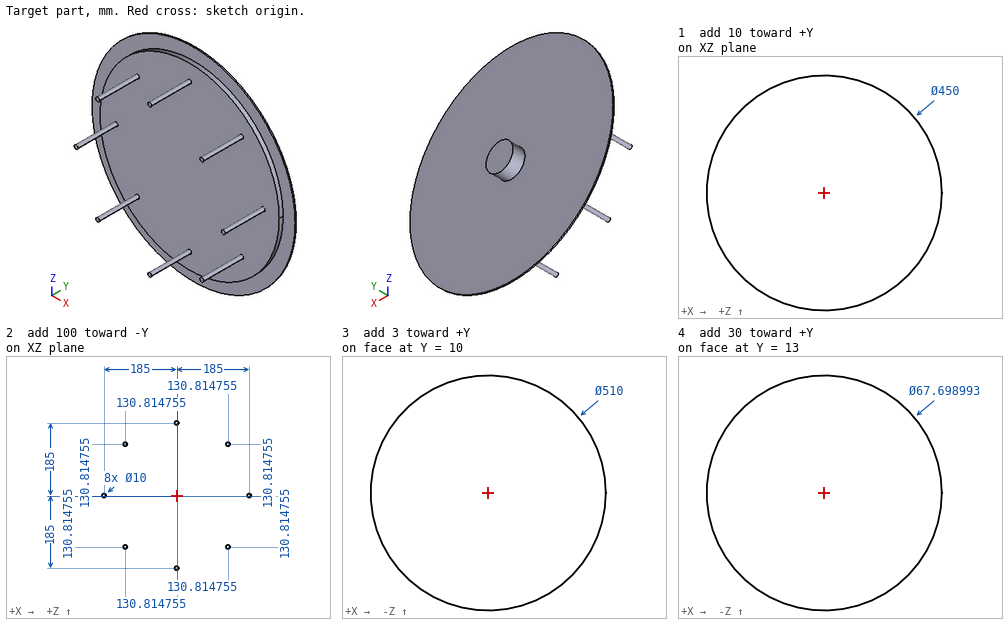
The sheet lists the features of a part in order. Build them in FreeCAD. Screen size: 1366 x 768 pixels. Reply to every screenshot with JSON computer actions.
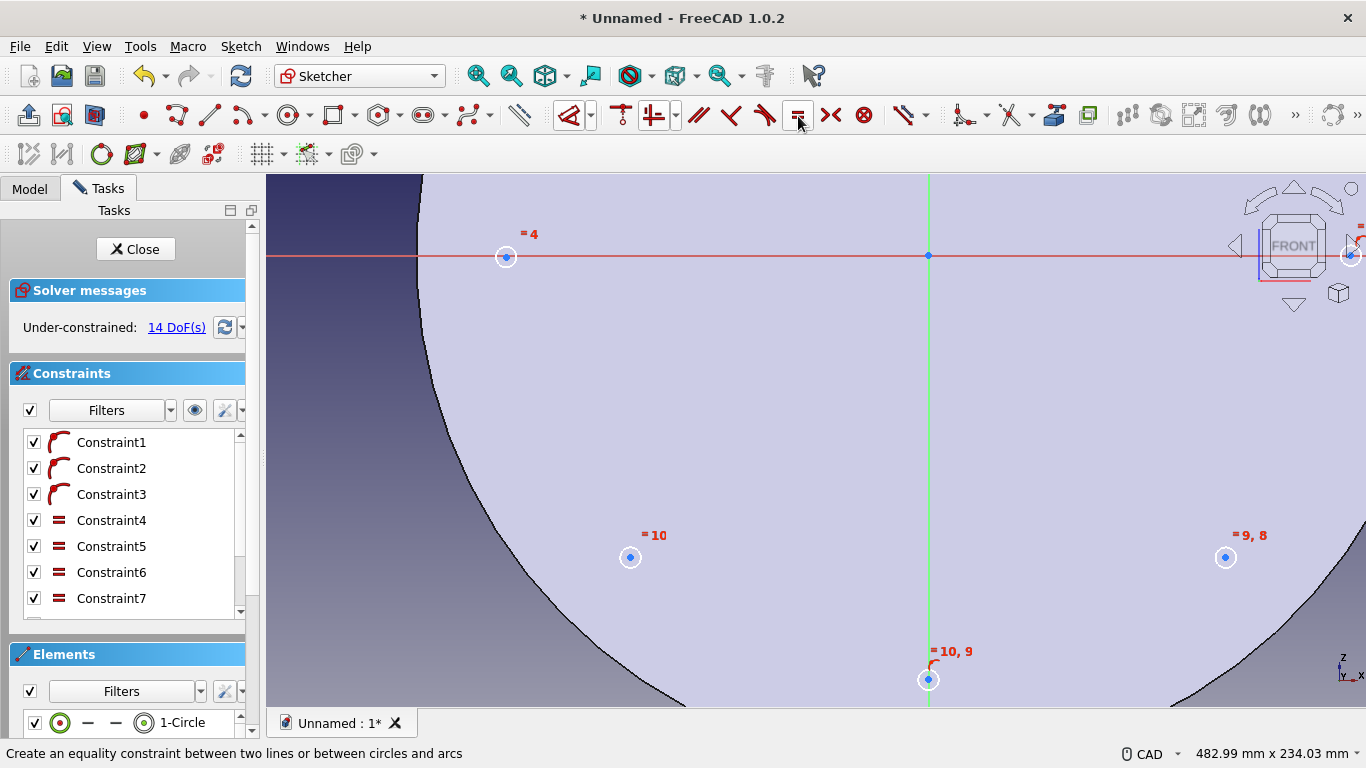
{"action": "left_click", "coordinate": [506, 257]}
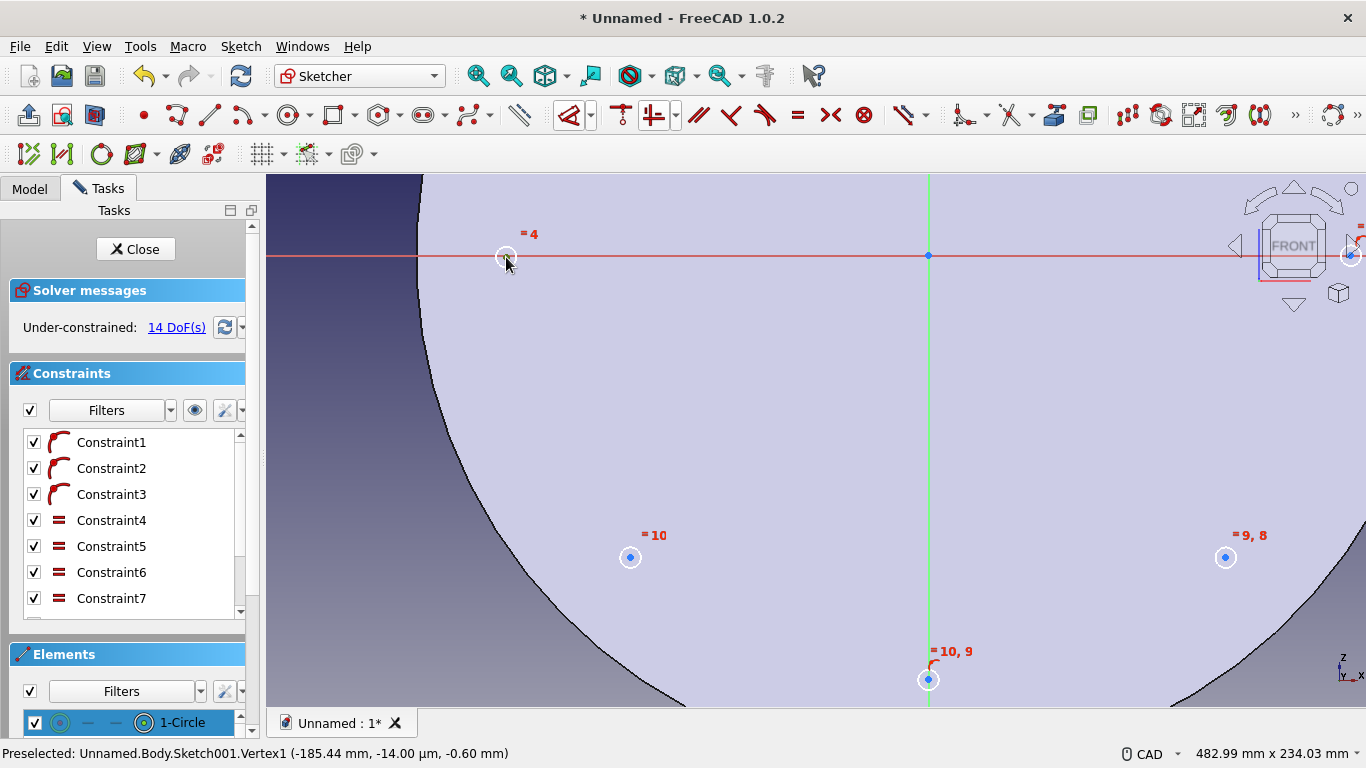
{"action": "left_click", "coordinate": [359, 256]}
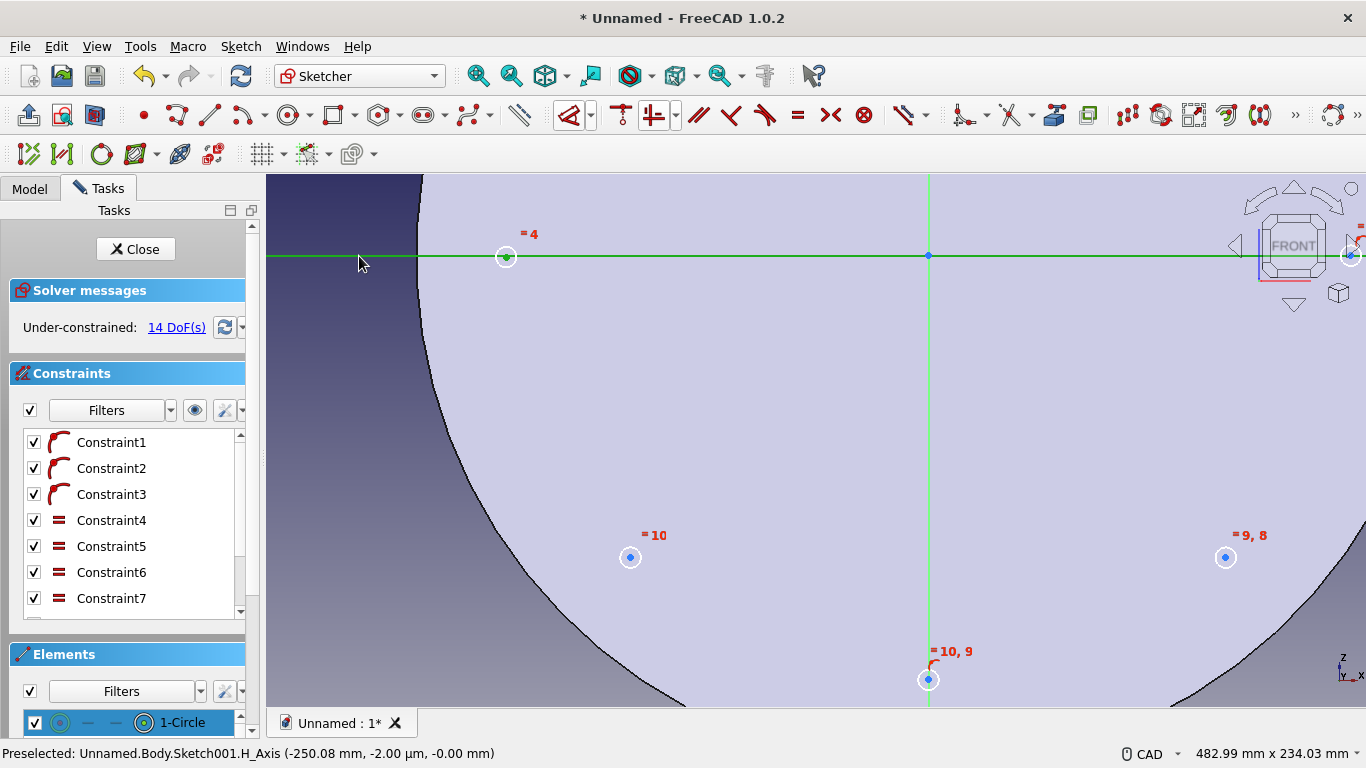
{"action": "left_click", "coordinate": [621, 116]}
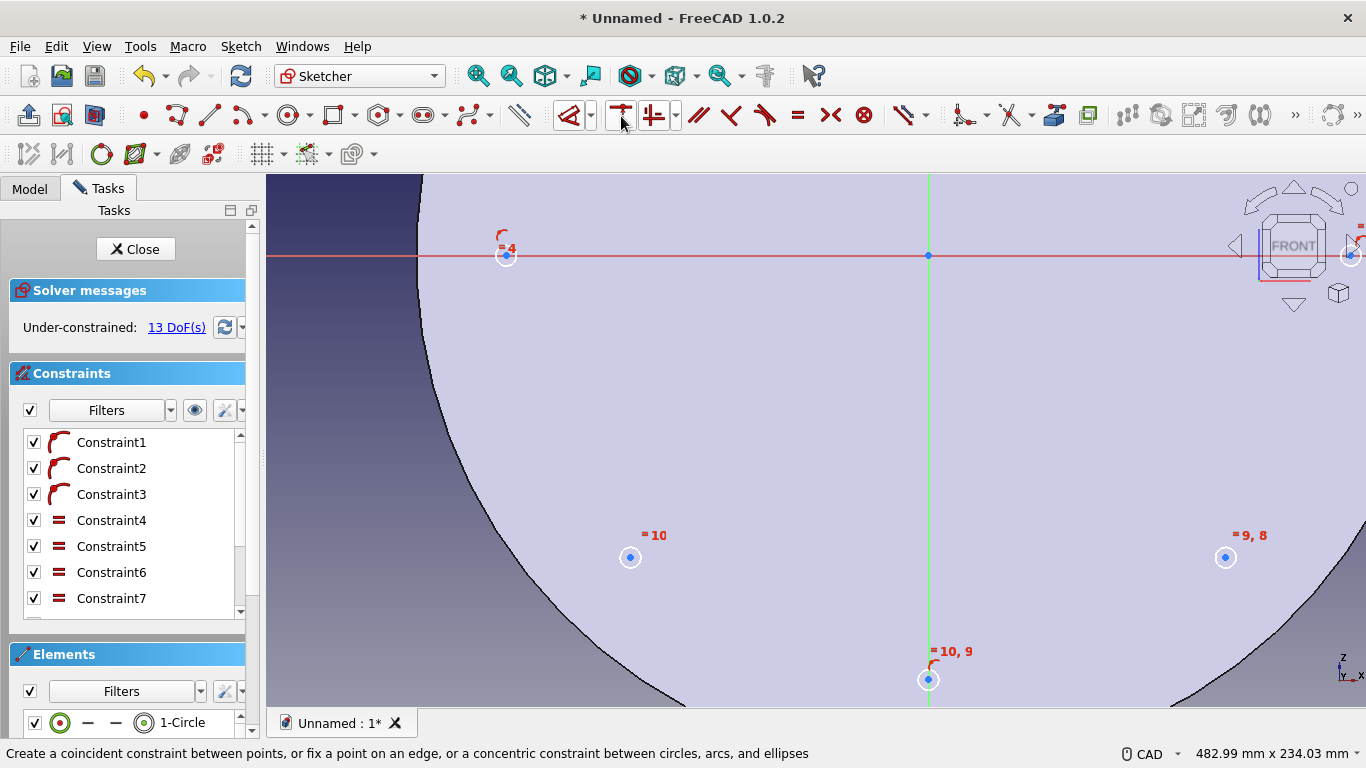
{"action": "scroll", "coordinate": [507, 245], "scroll_direction": "up", "scroll_amount": 3}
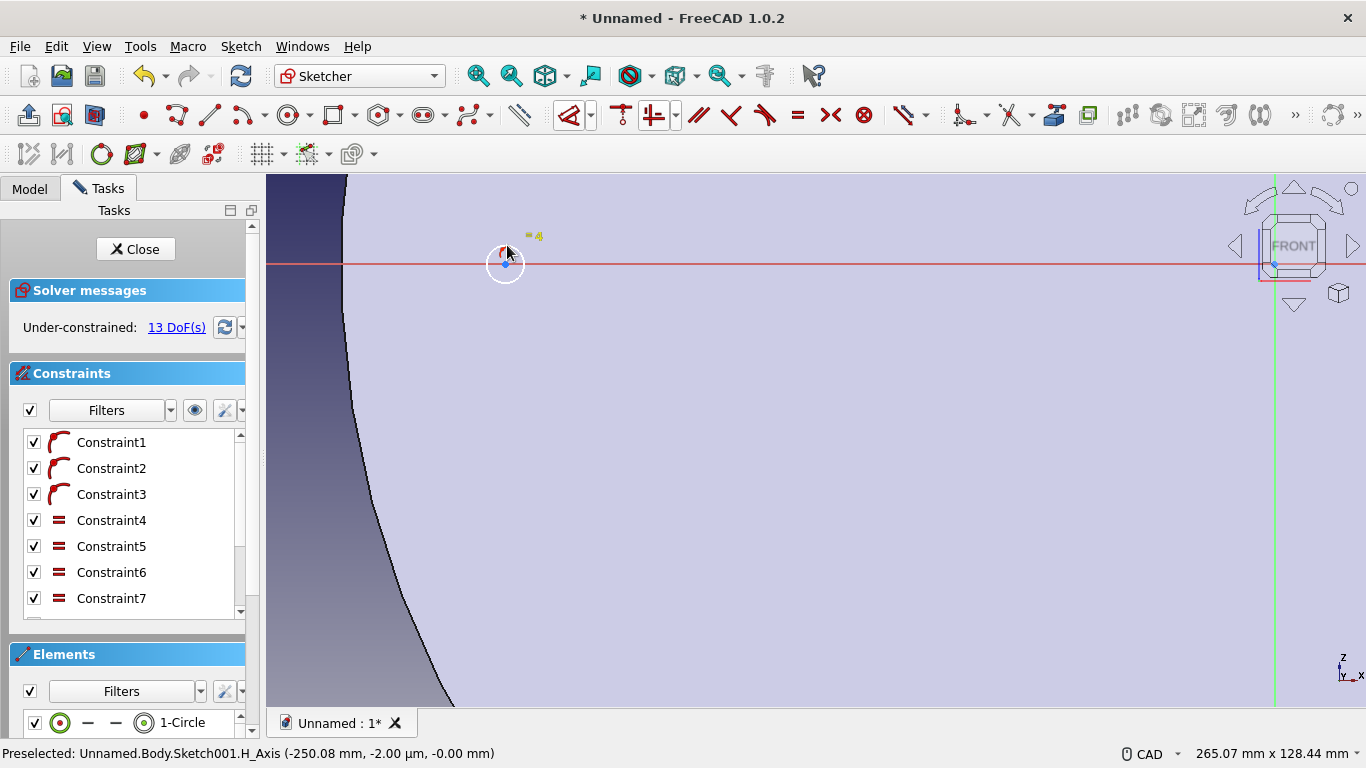
{"action": "left_click", "coordinate": [487, 264]}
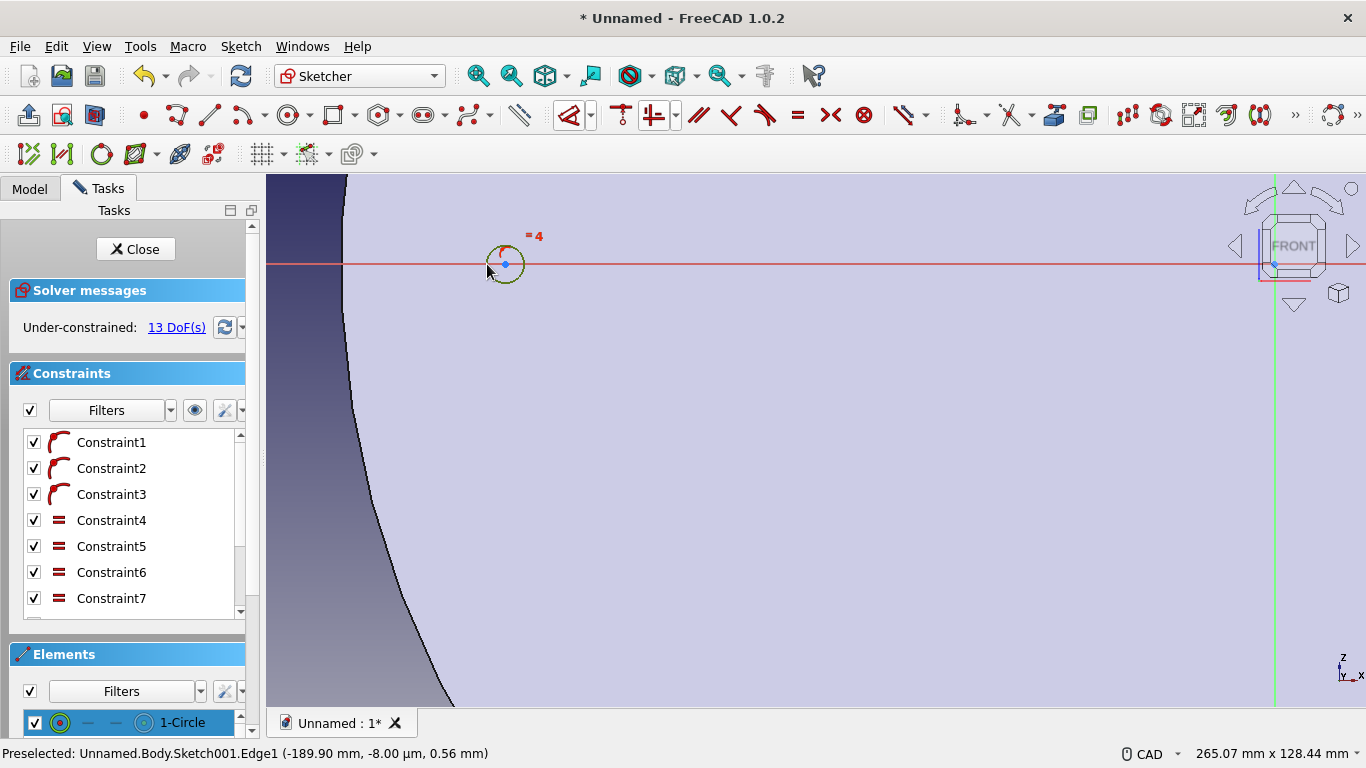
{"action": "key", "text": "k o"}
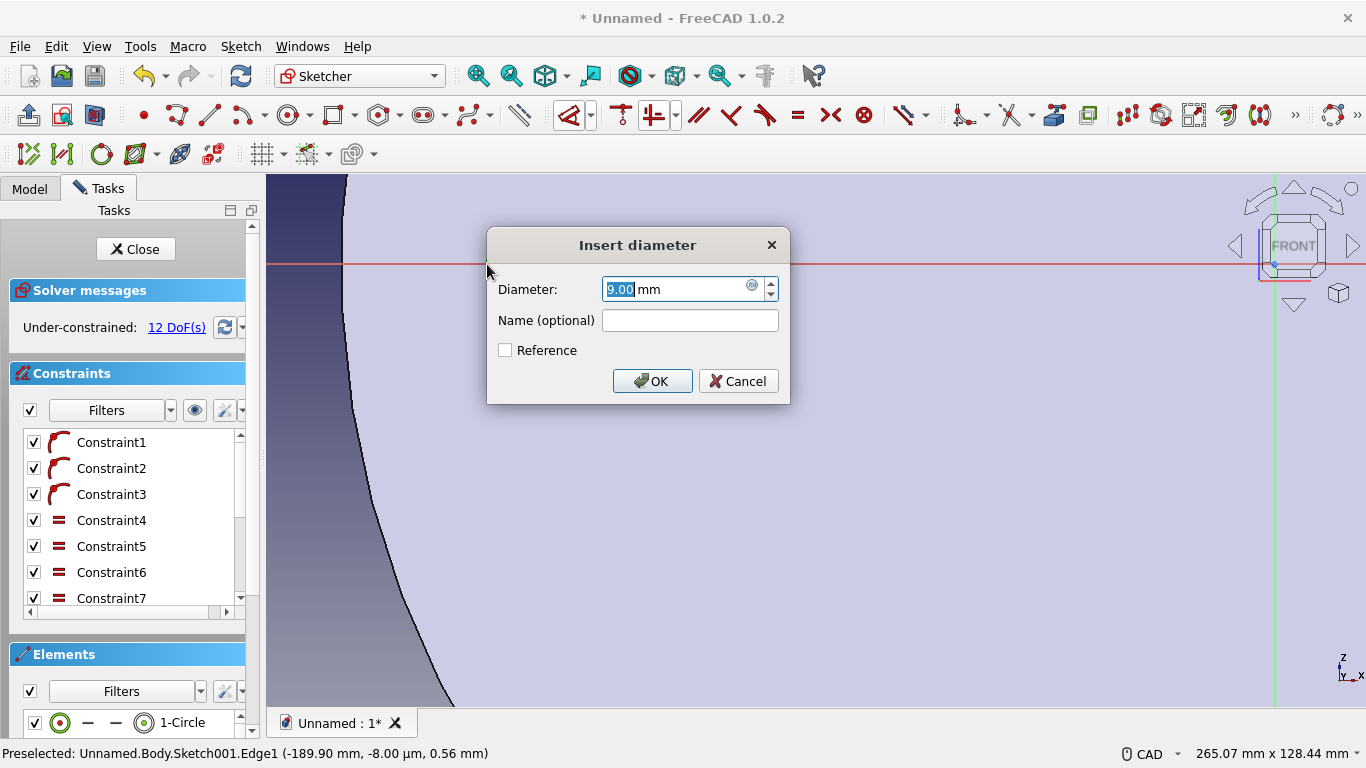
{"action": "type", "text": "10"}
{"action": "key", "text": "Return"}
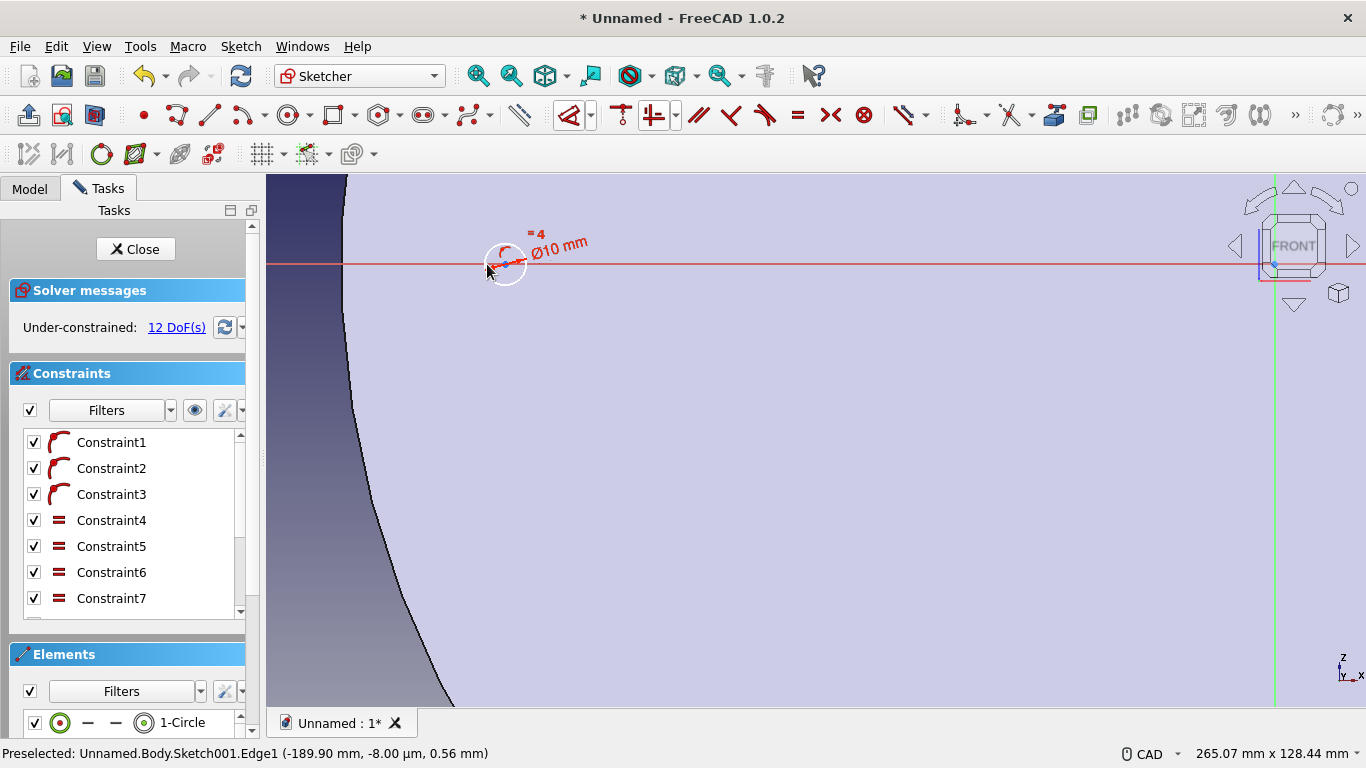
{"action": "scroll", "coordinate": [614, 485], "scroll_direction": "down", "scroll_amount": 8}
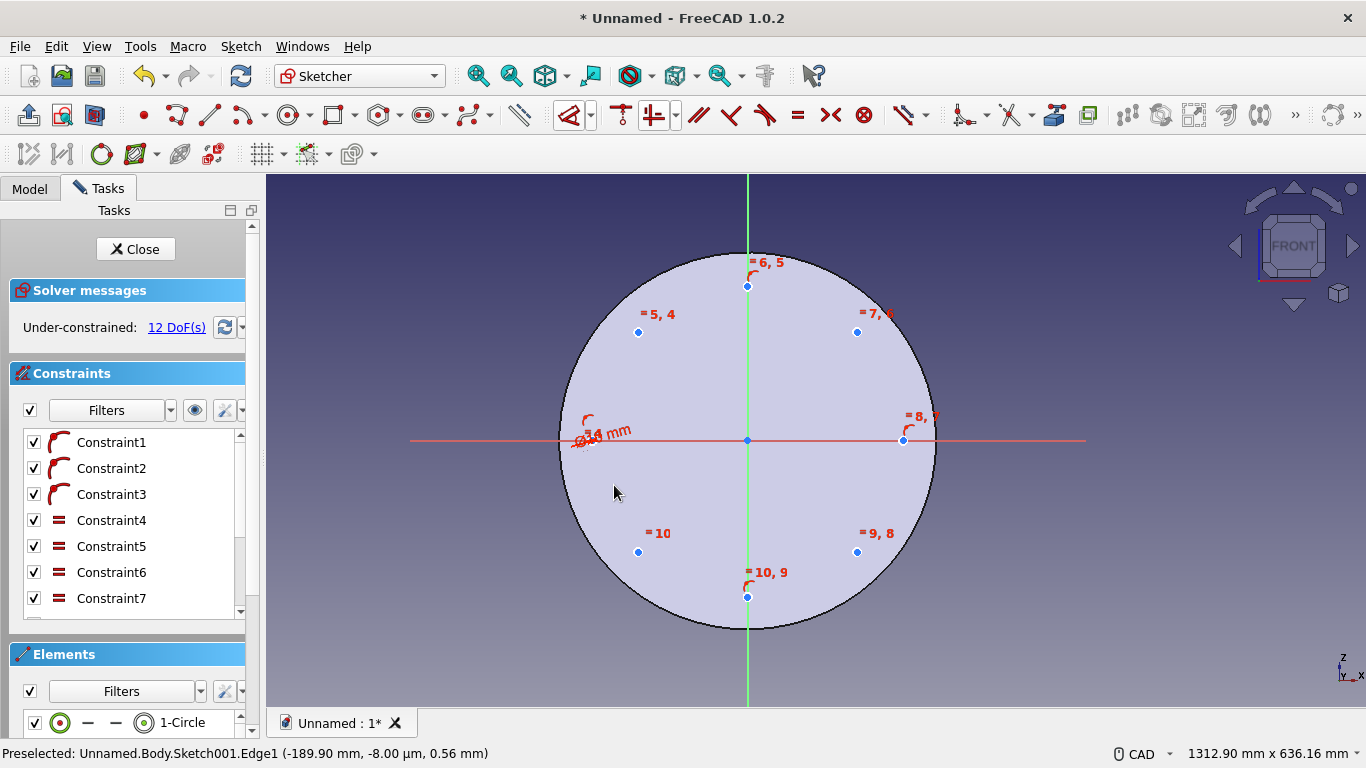
{"action": "left_click", "coordinate": [592, 441]}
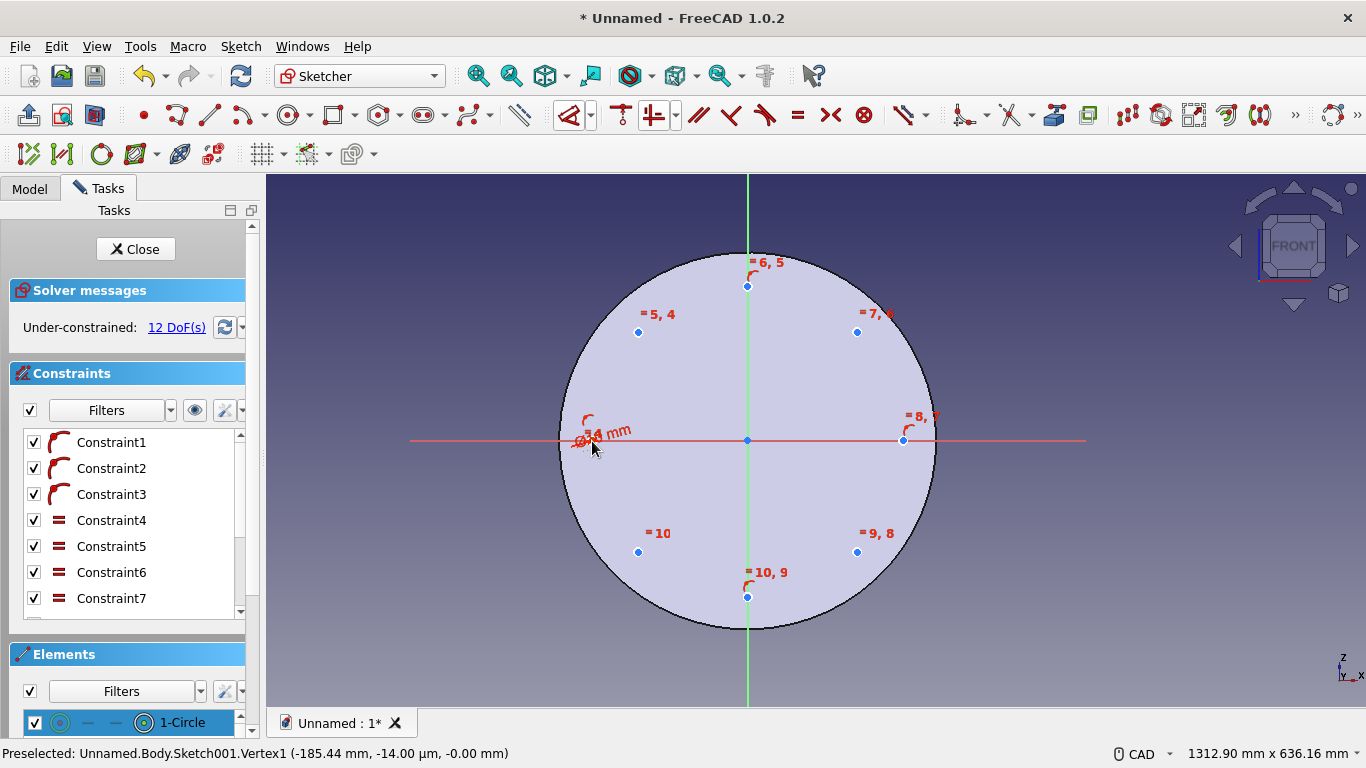
{"action": "left_click", "coordinate": [590, 116]}